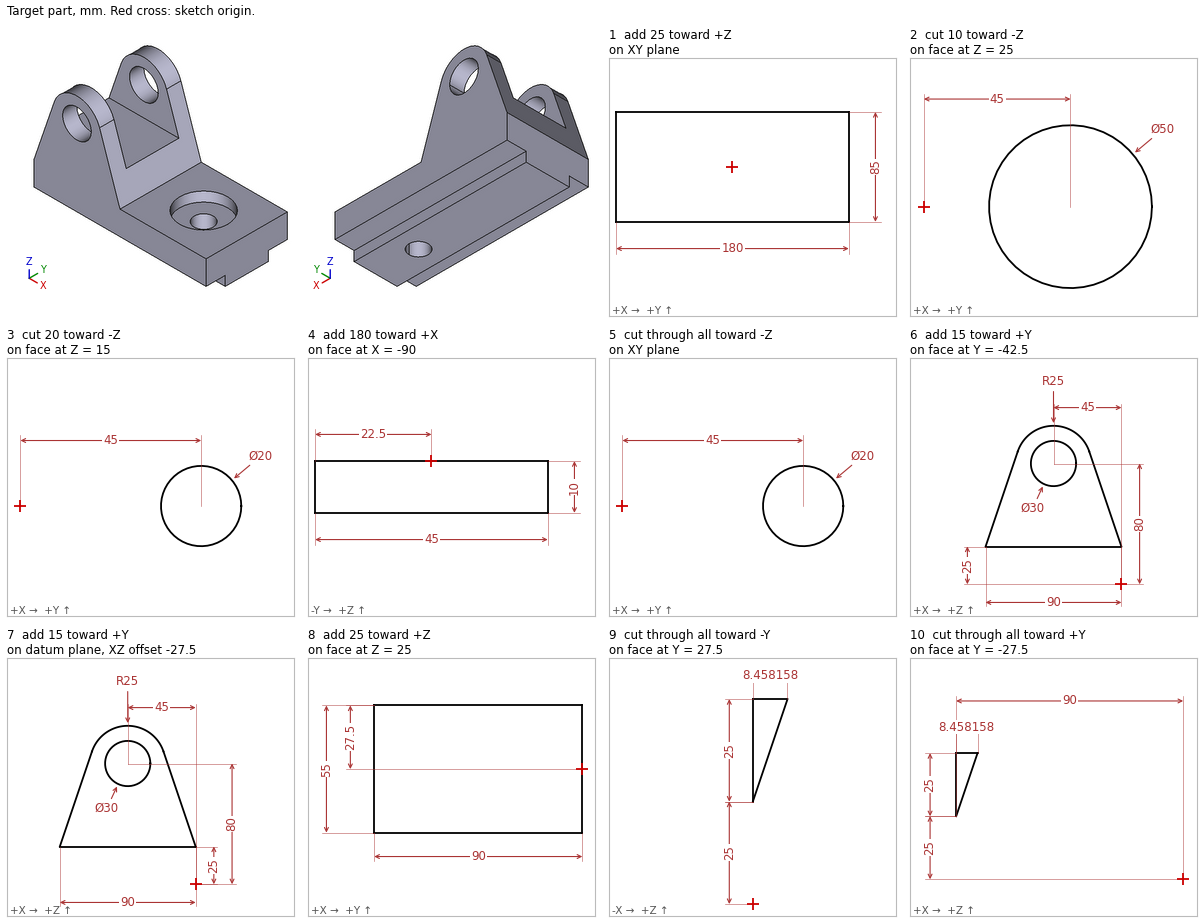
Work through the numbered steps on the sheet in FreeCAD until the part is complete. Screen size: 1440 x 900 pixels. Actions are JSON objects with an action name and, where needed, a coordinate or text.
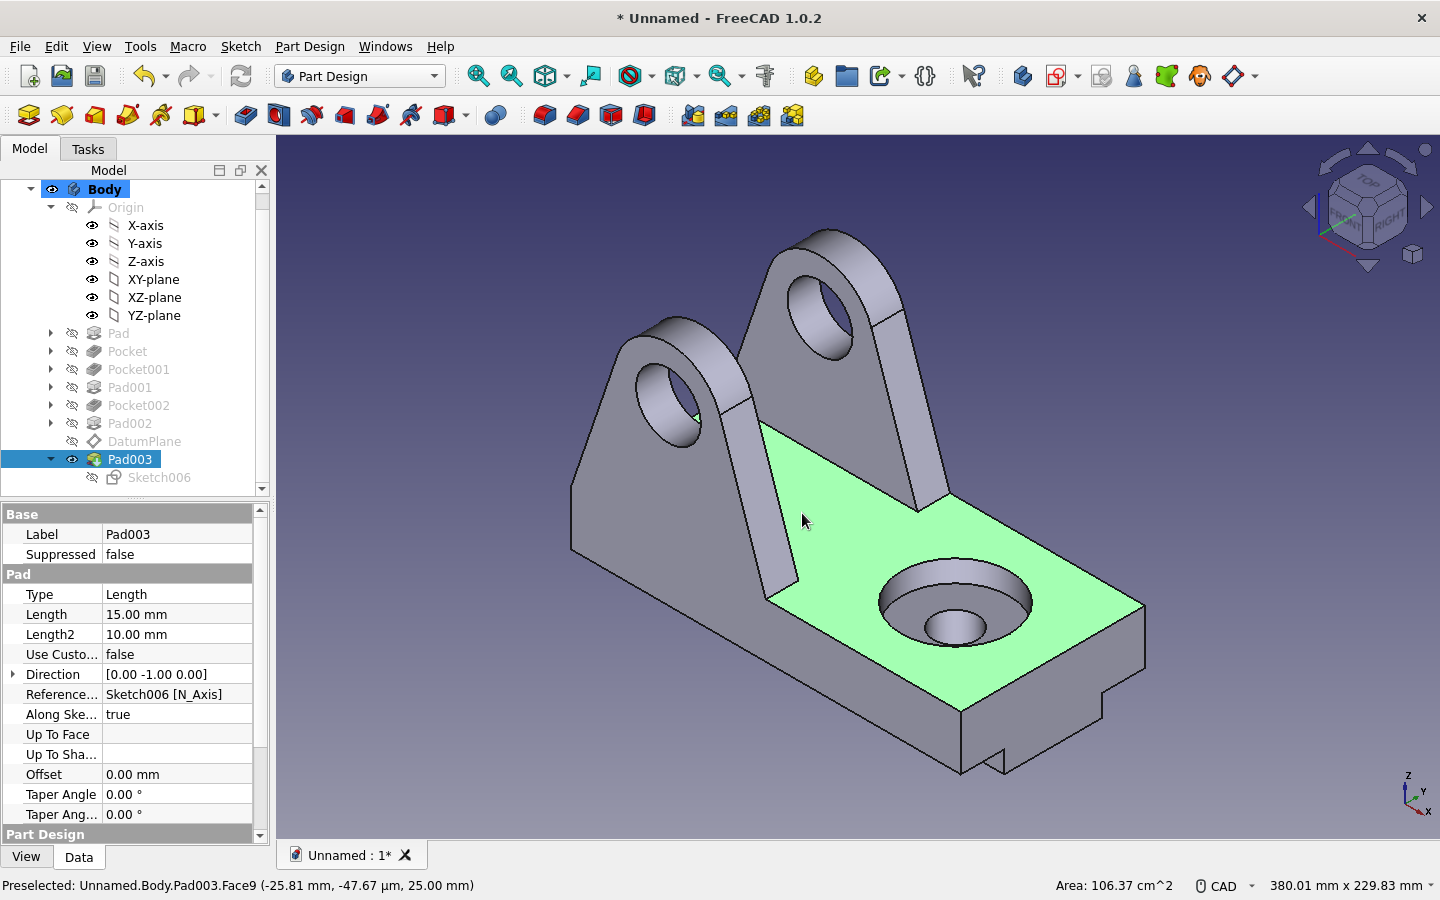
{"action": "left_click", "coordinate": [1056, 76]}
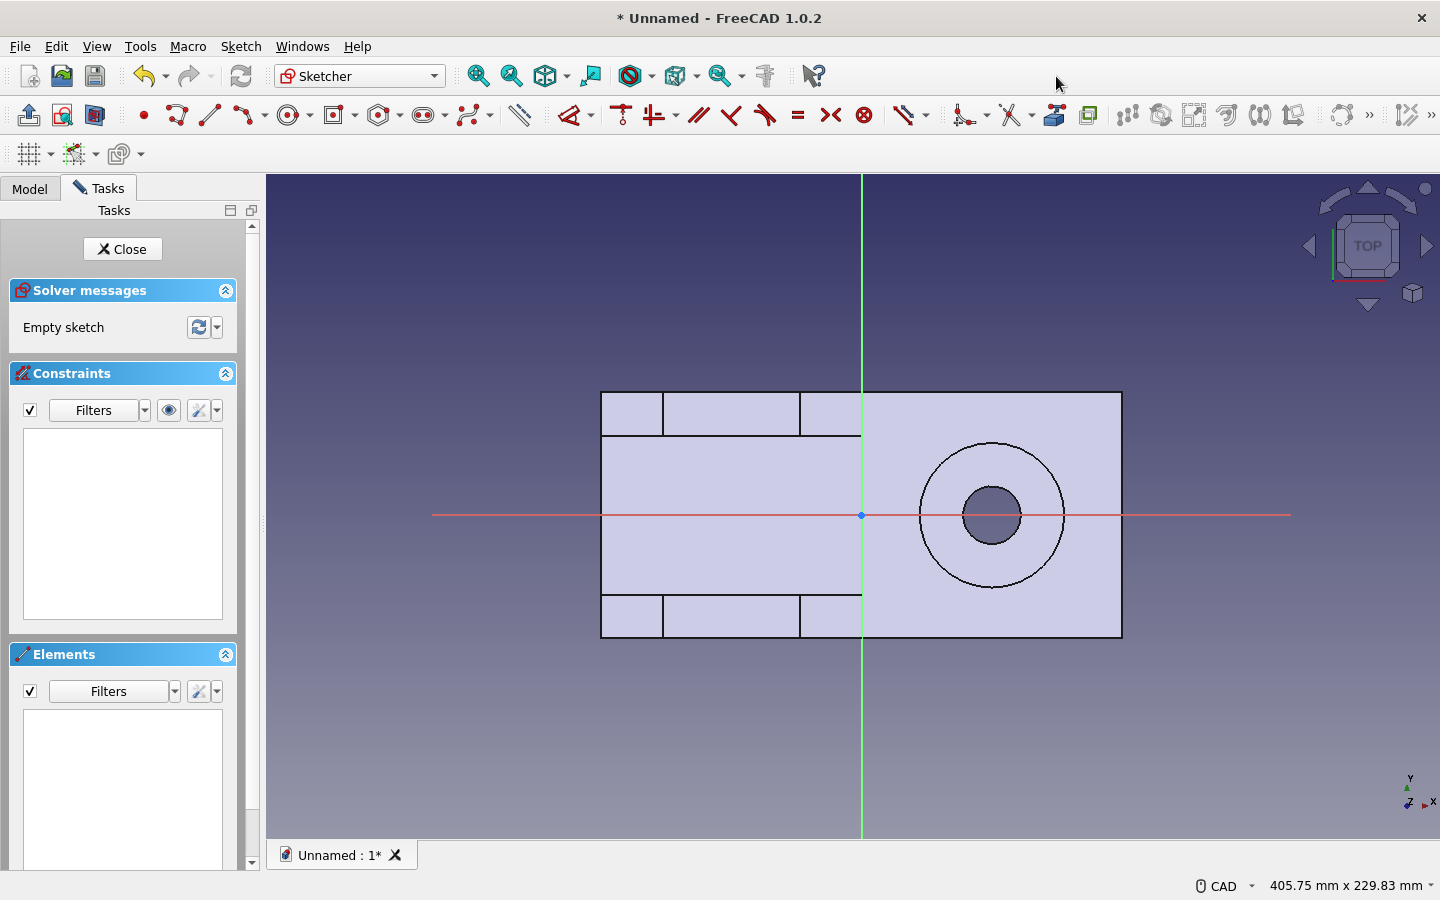
{"action": "scroll", "coordinate": [701, 520], "scroll_direction": "up", "scroll_amount": 5}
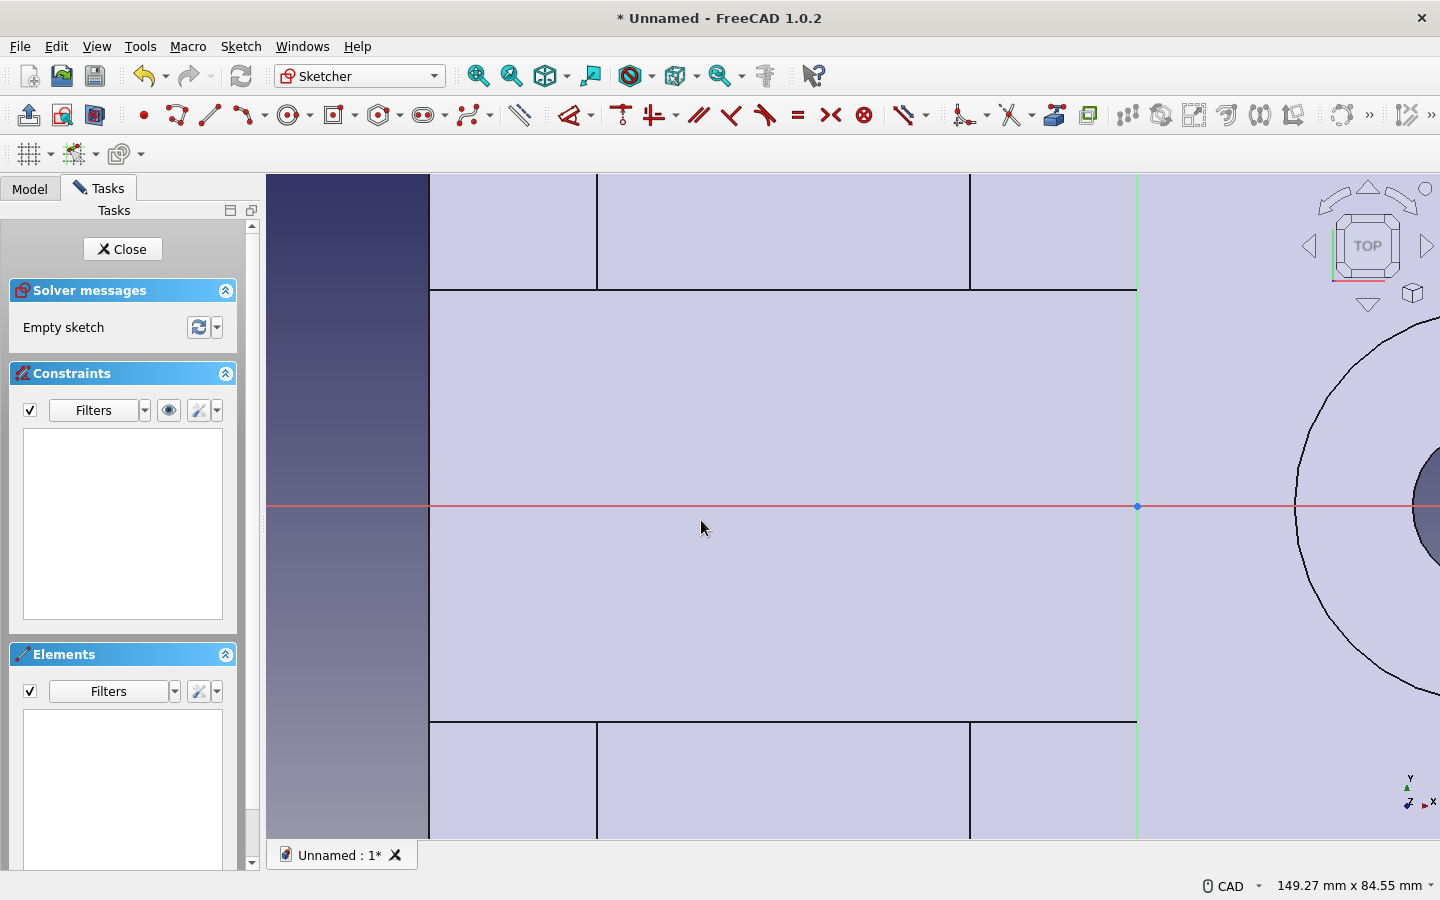
{"action": "left_click", "coordinate": [354, 116]}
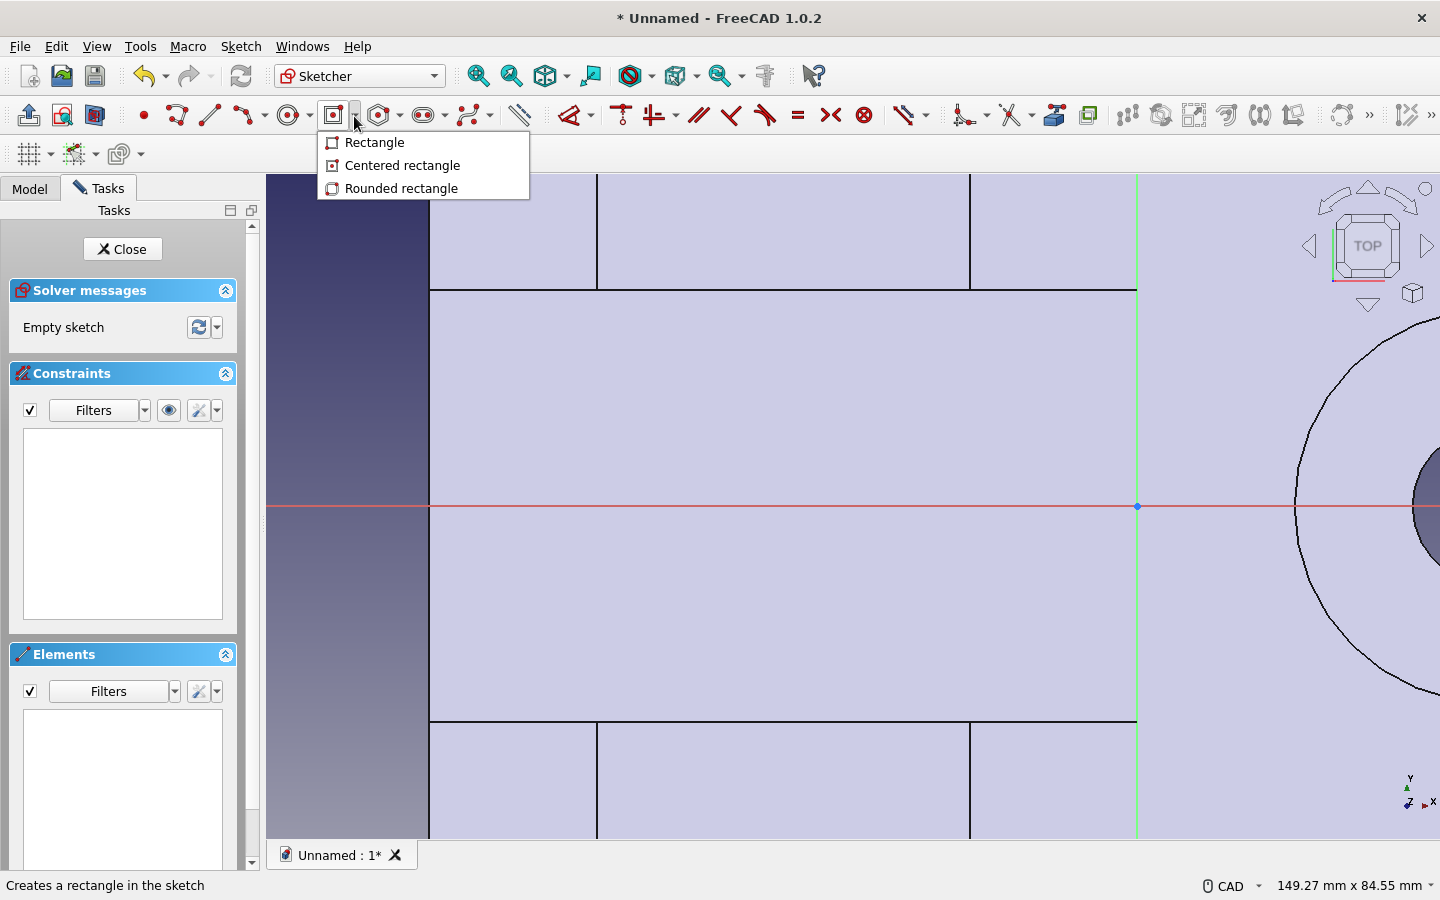
{"action": "left_click", "coordinate": [424, 142]}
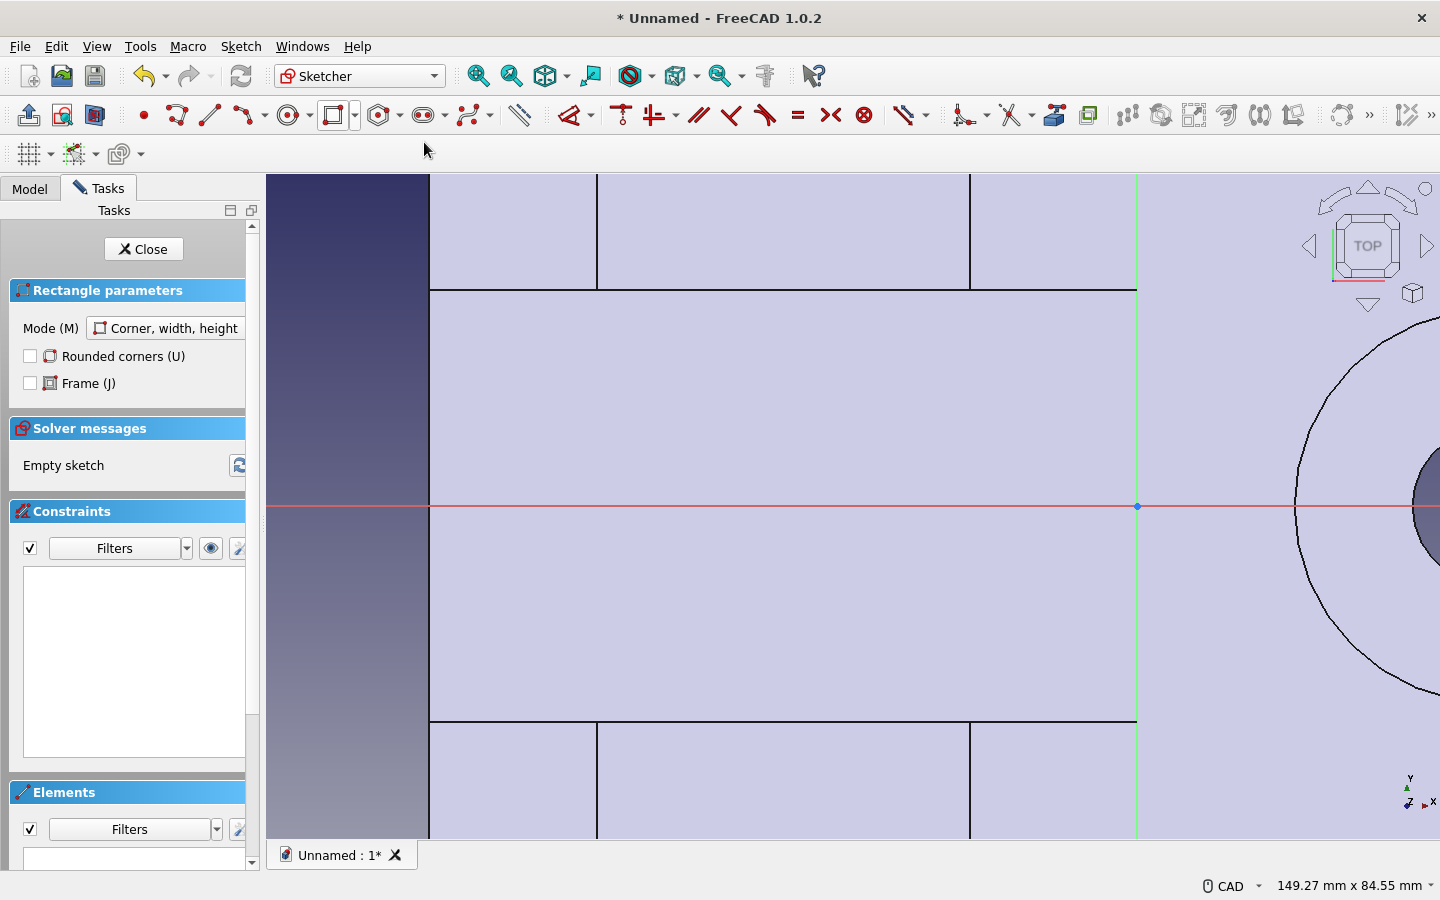
{"action": "left_click", "coordinate": [429, 290]}
{"action": "left_click", "coordinate": [1137, 722]}
{"action": "key", "text": "Escape"}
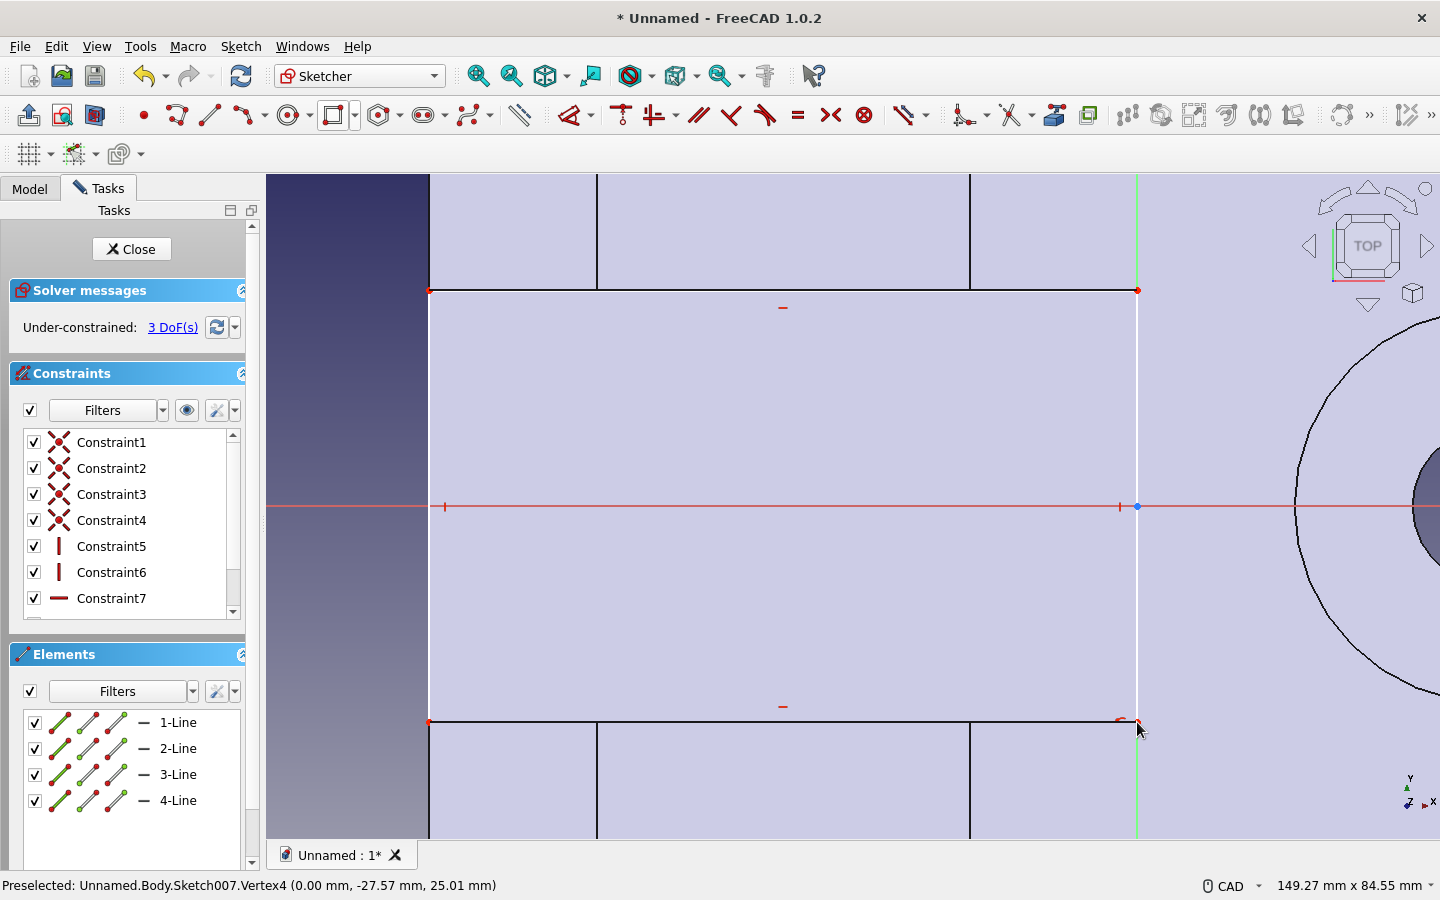
{"action": "left_click", "coordinate": [568, 116]}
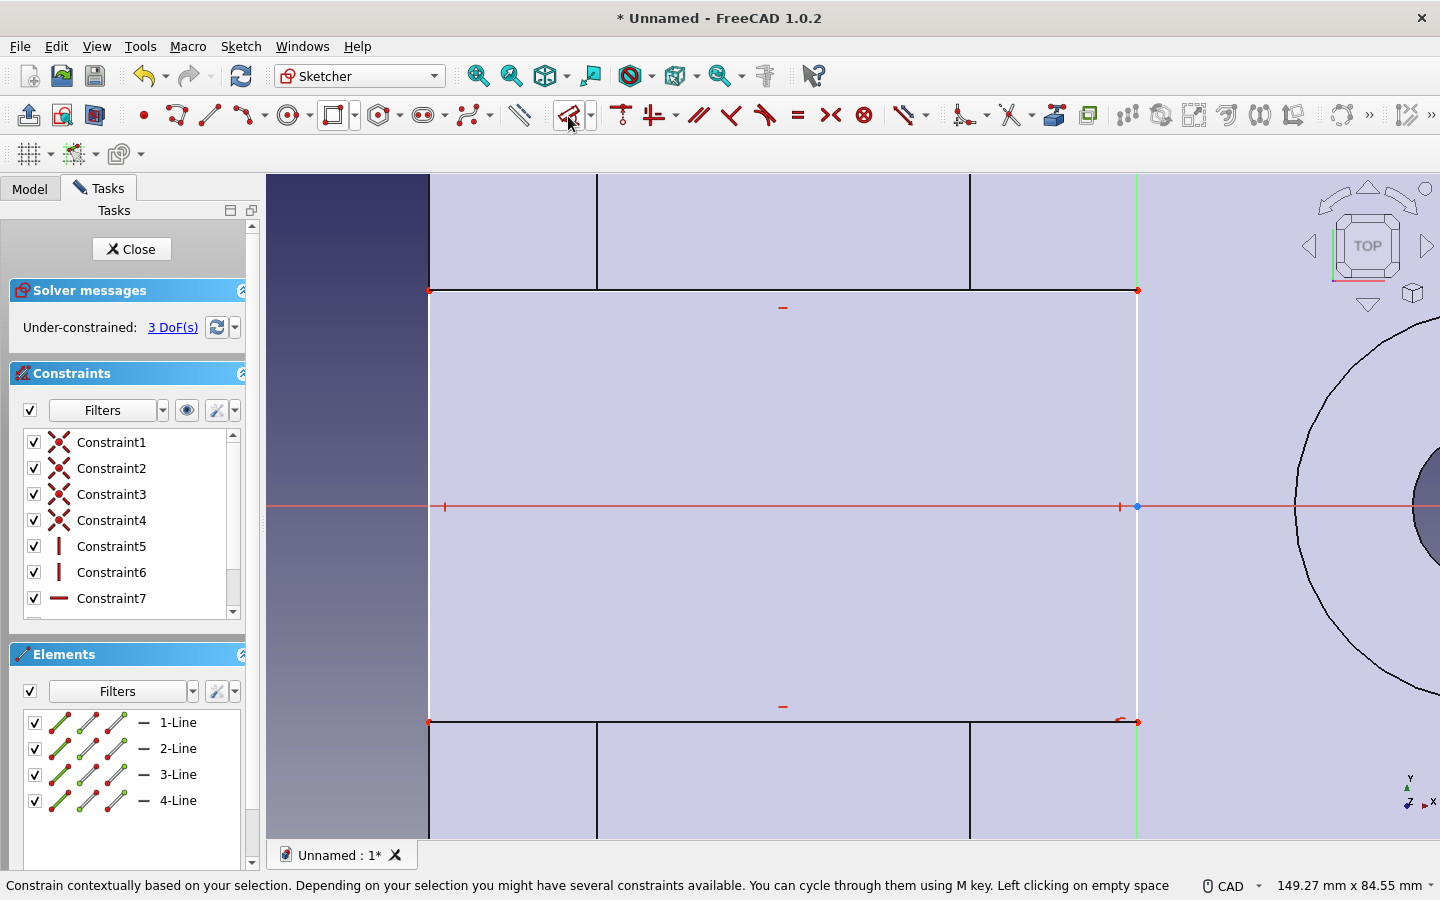
{"action": "left_click", "coordinate": [429, 421]}
{"action": "left_click", "coordinate": [395, 408]}